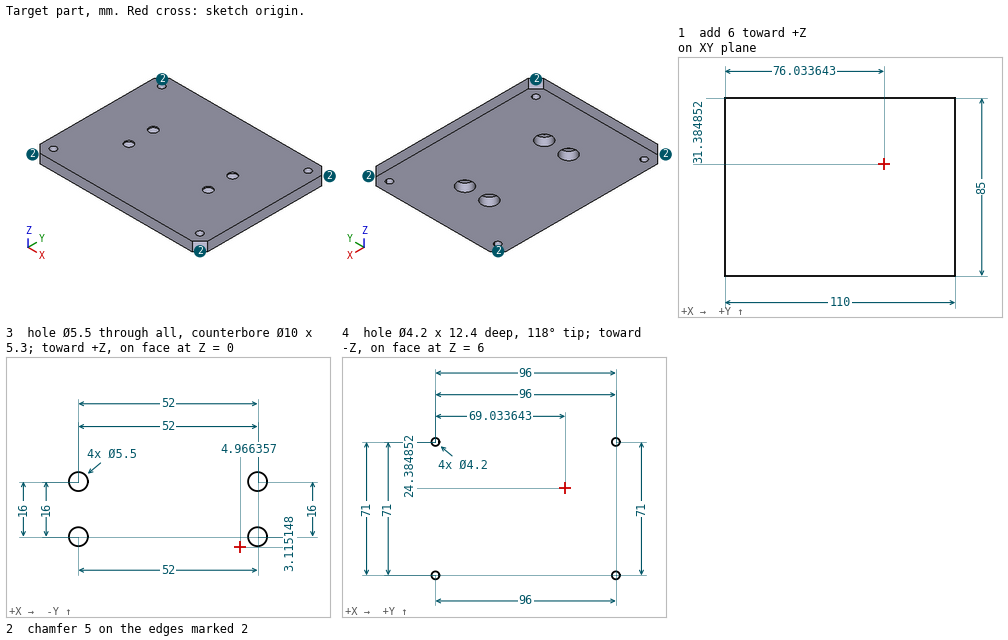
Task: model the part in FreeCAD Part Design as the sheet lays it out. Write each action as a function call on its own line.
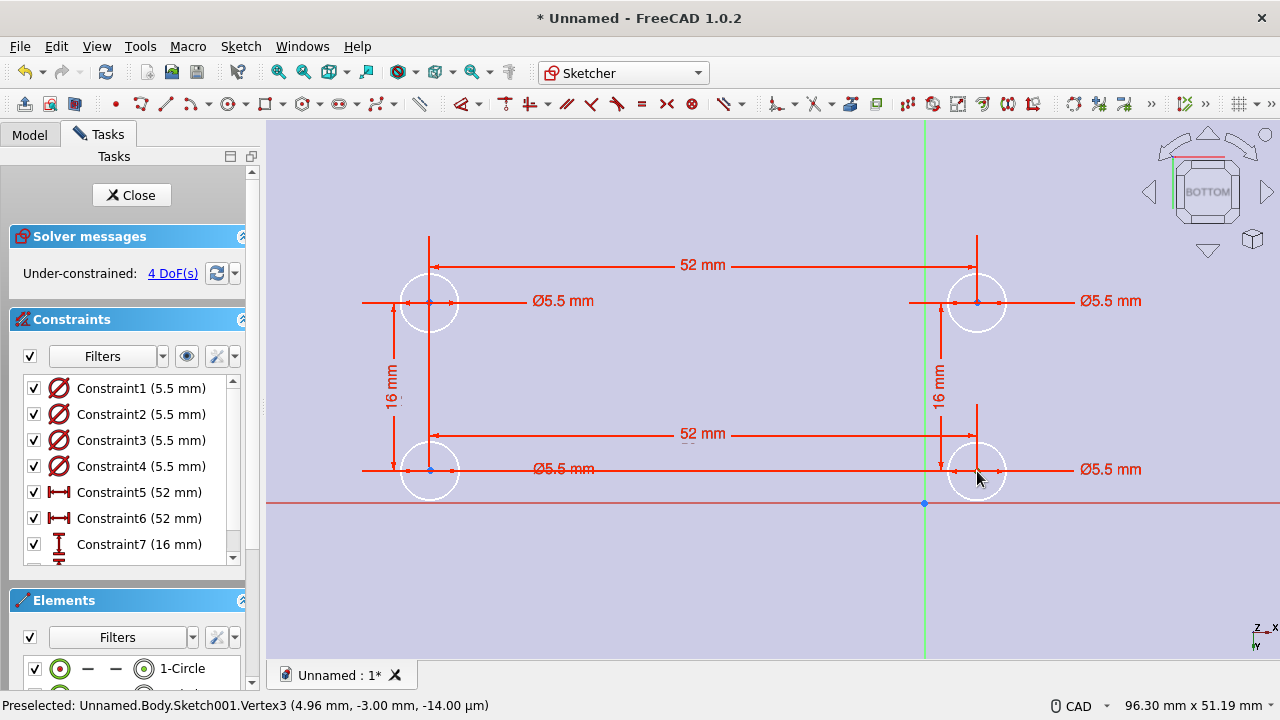
click(430, 471)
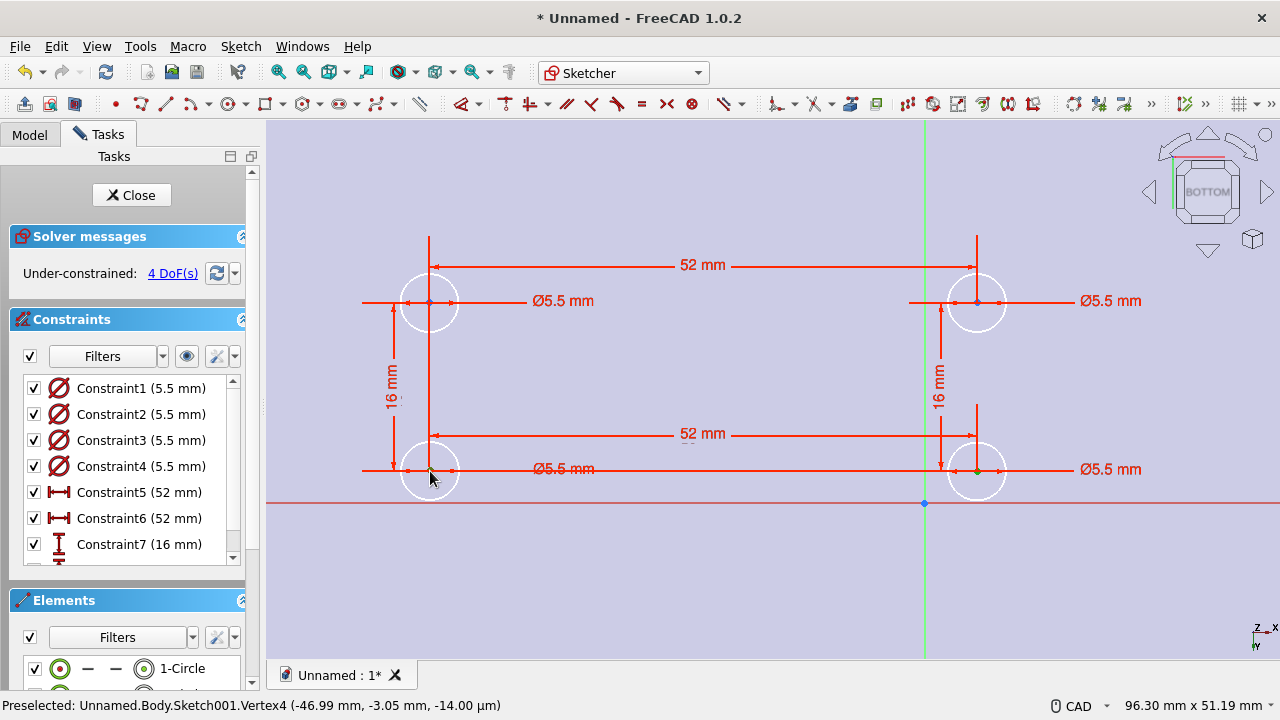
click(478, 104)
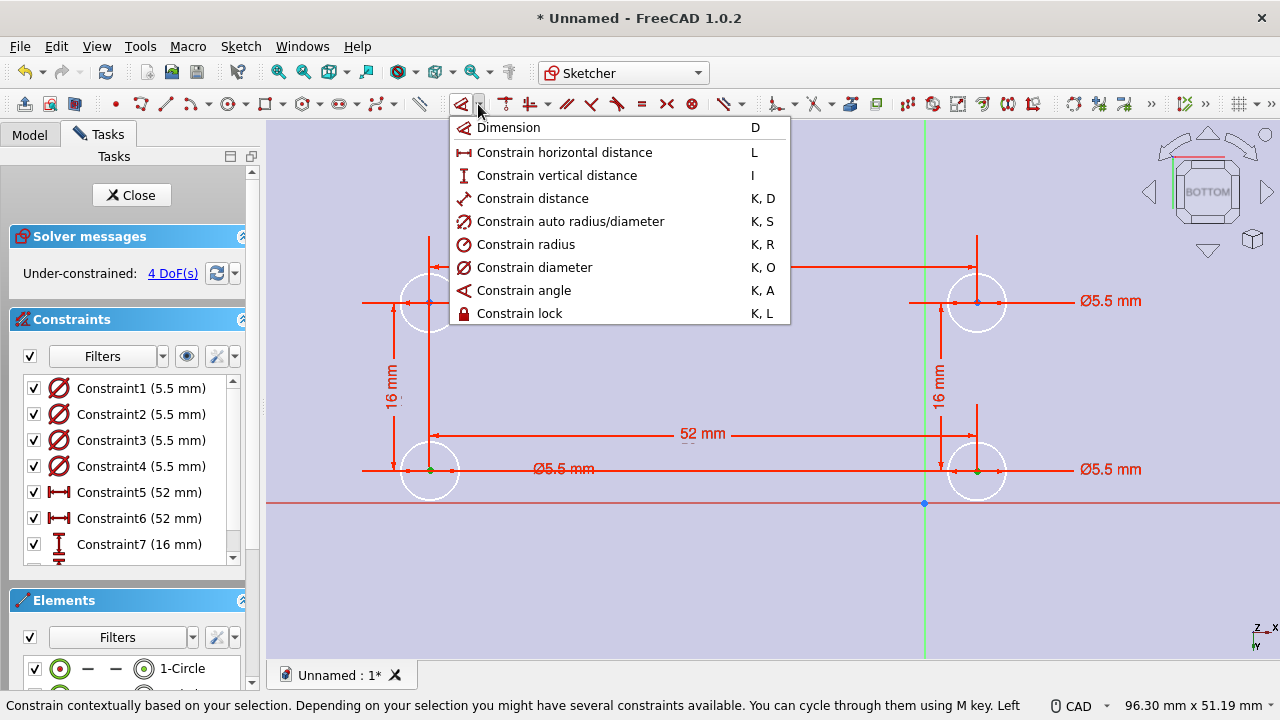
click(620, 152)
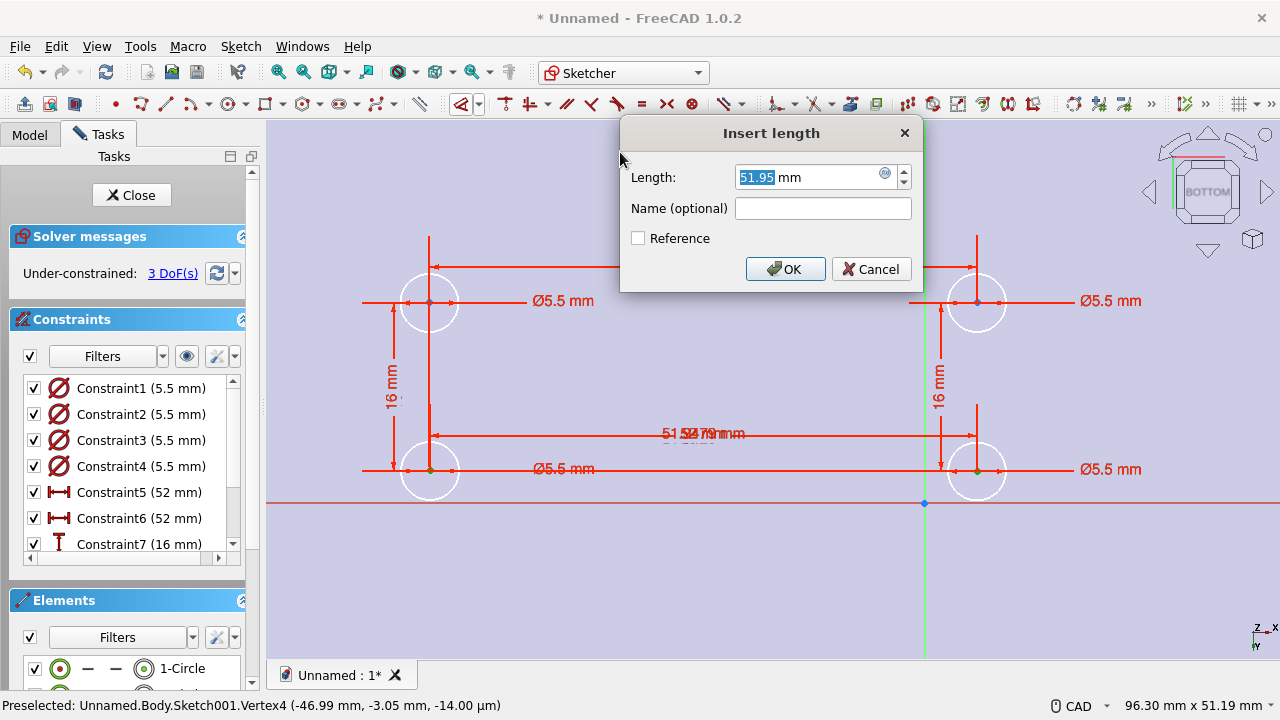
text(52)
key(Return)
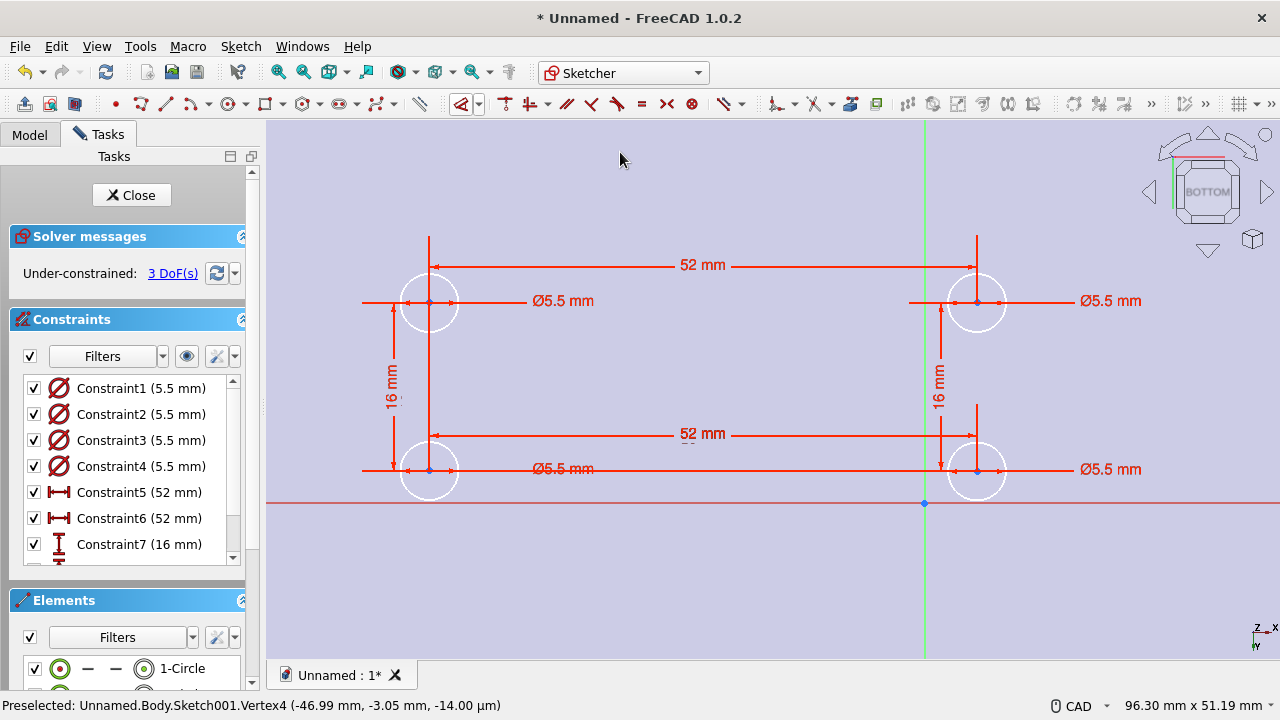
click(429, 303)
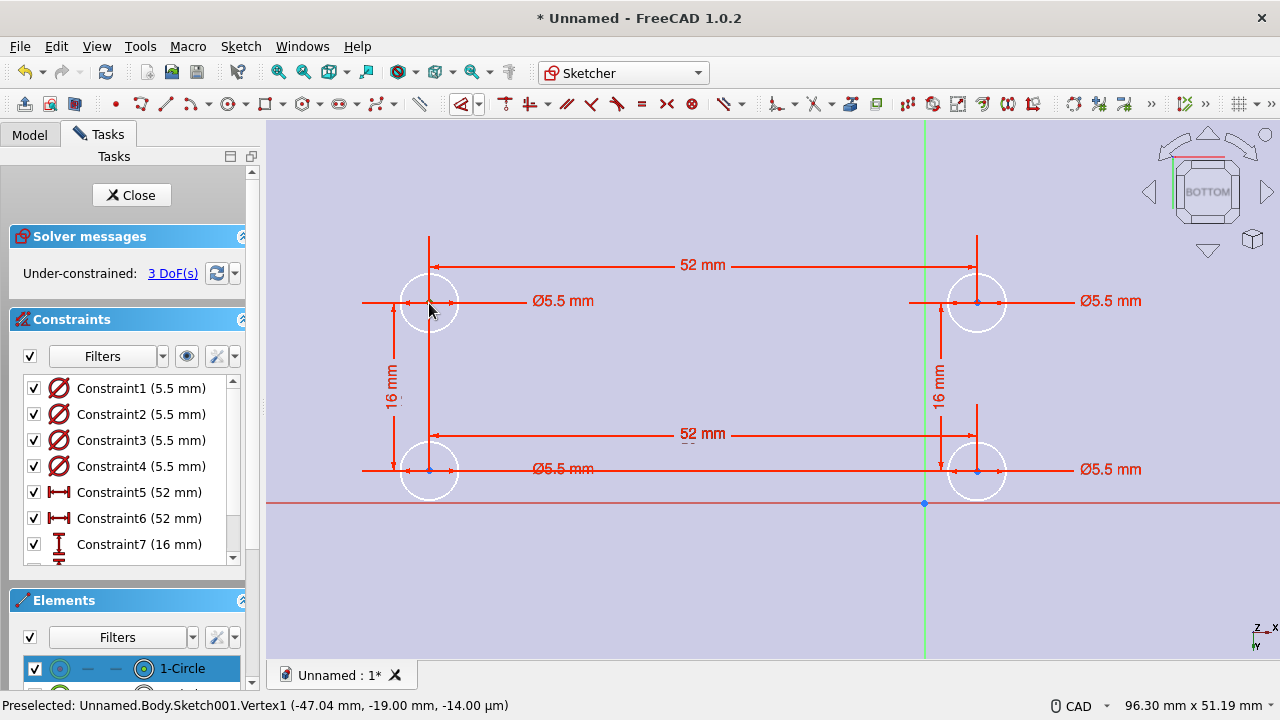
click(429, 471)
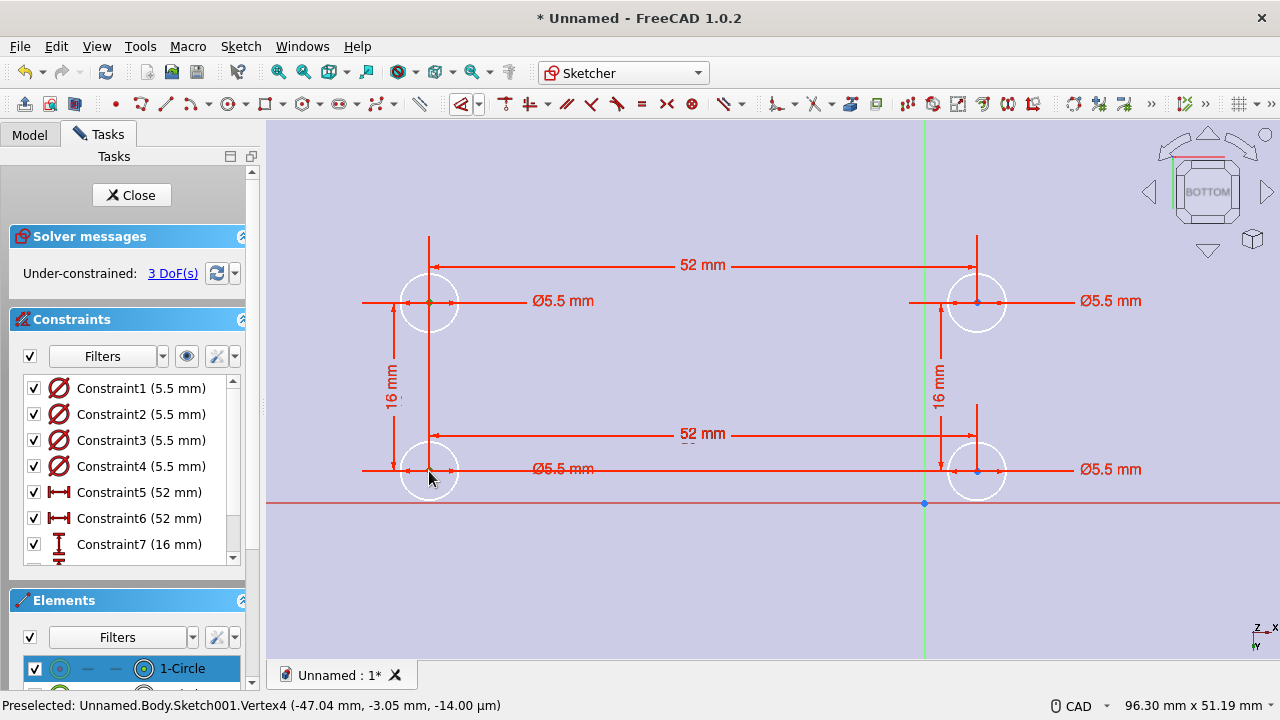
key(i)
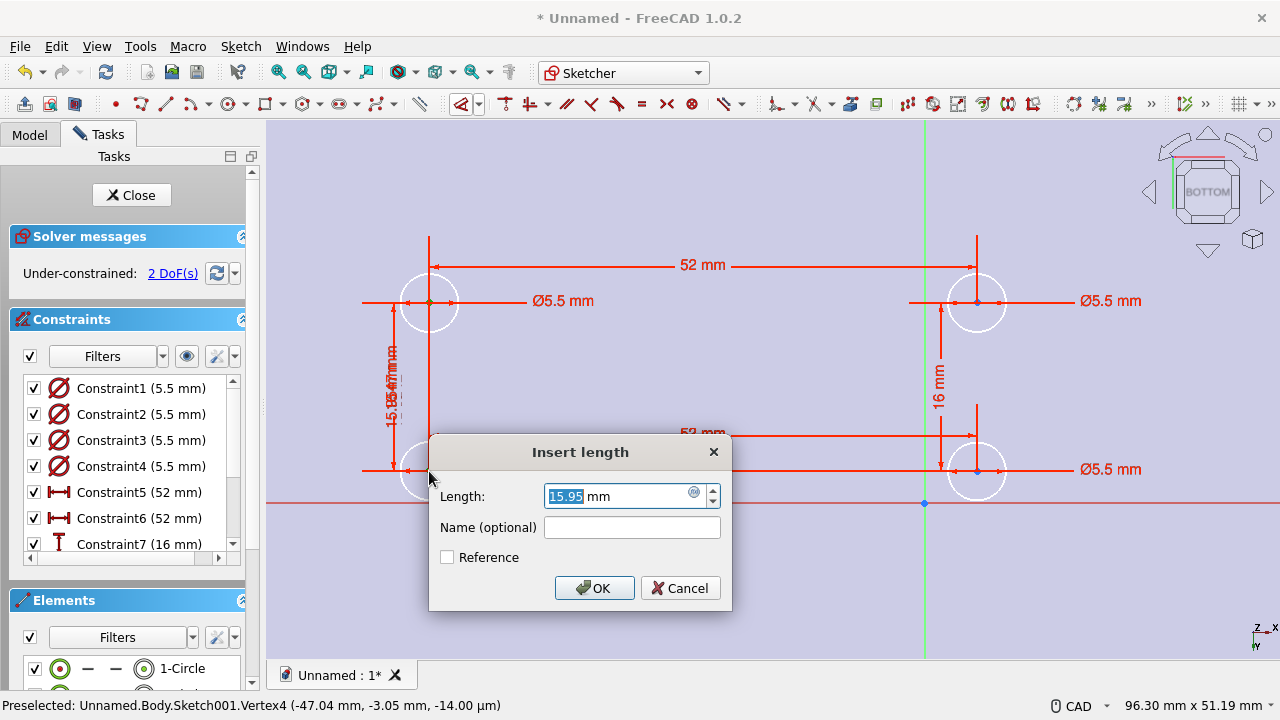
text(16)
key(Return)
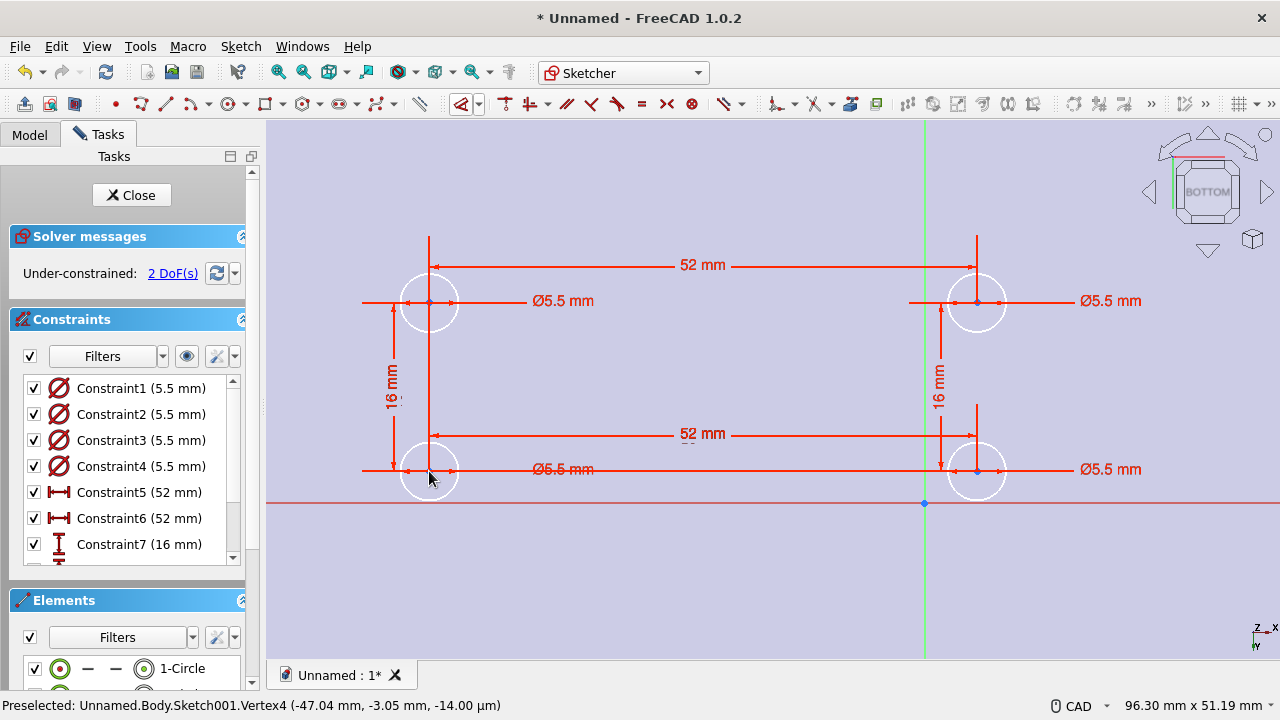
click(977, 303)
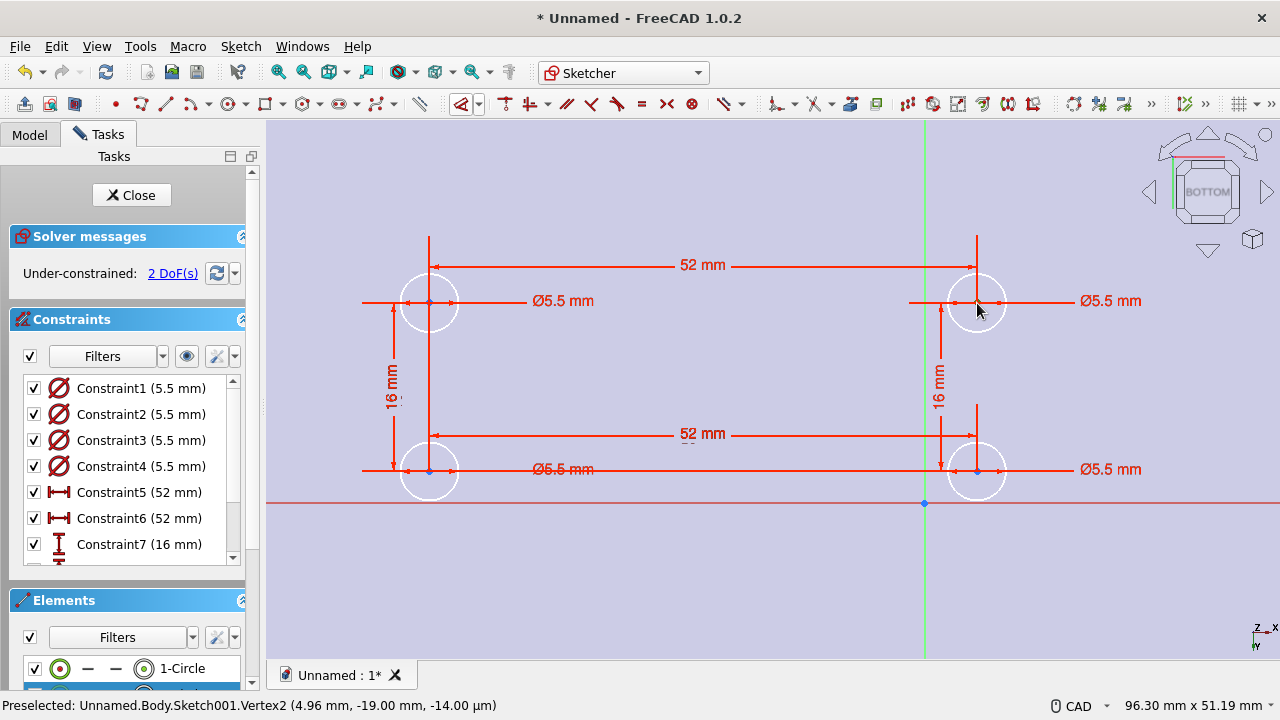
key(l)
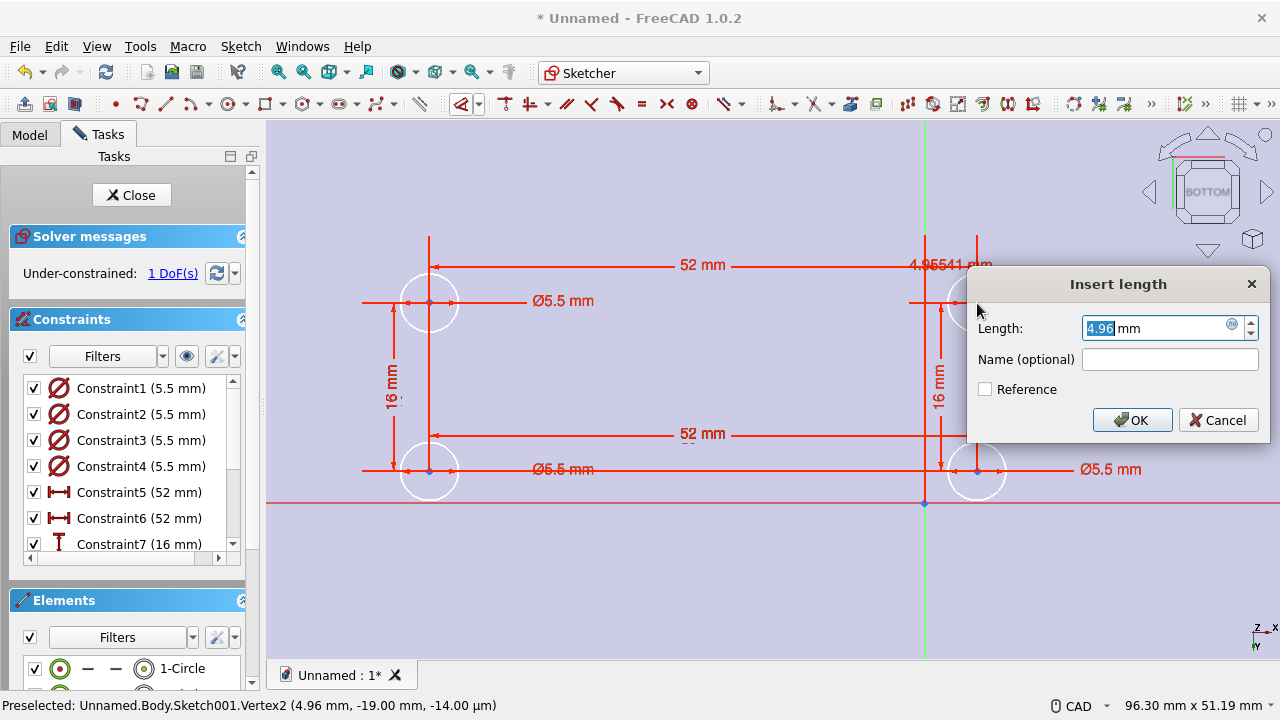
text(4.966357)
key(Return)